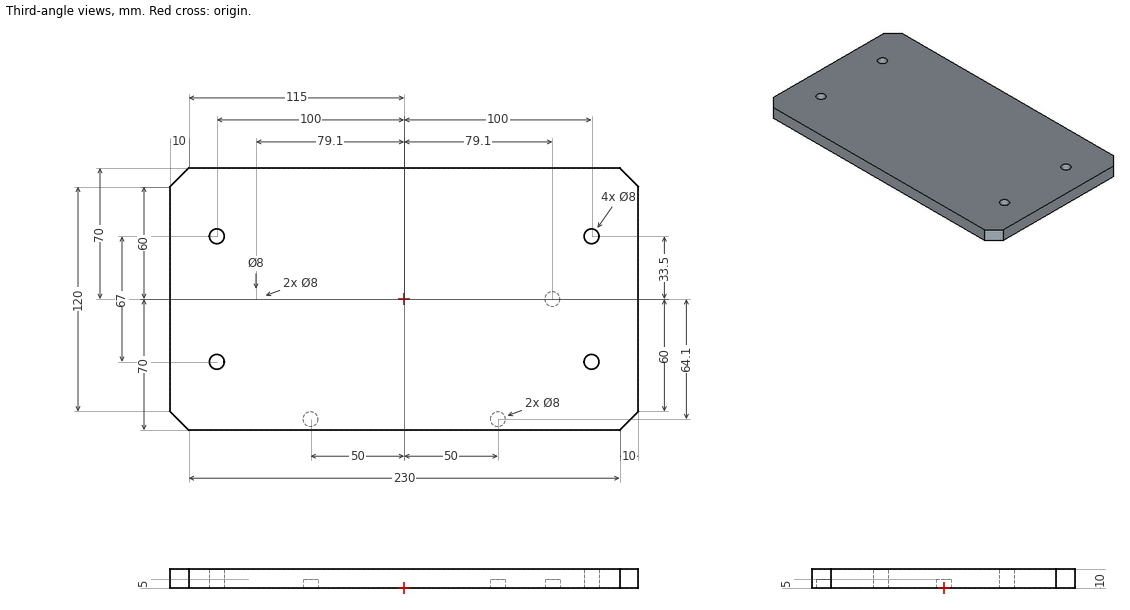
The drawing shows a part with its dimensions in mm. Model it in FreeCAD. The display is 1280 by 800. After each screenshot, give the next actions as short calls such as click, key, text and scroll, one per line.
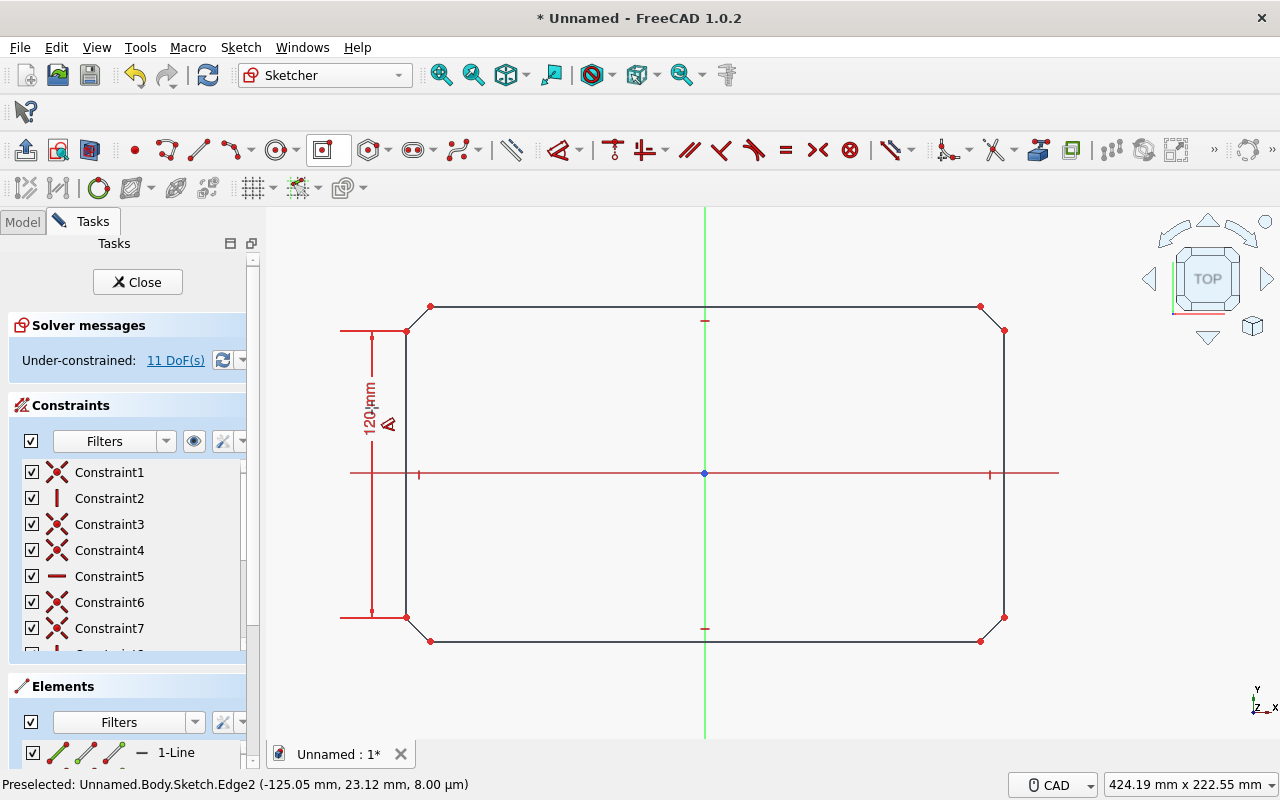
click(595, 642)
click(579, 676)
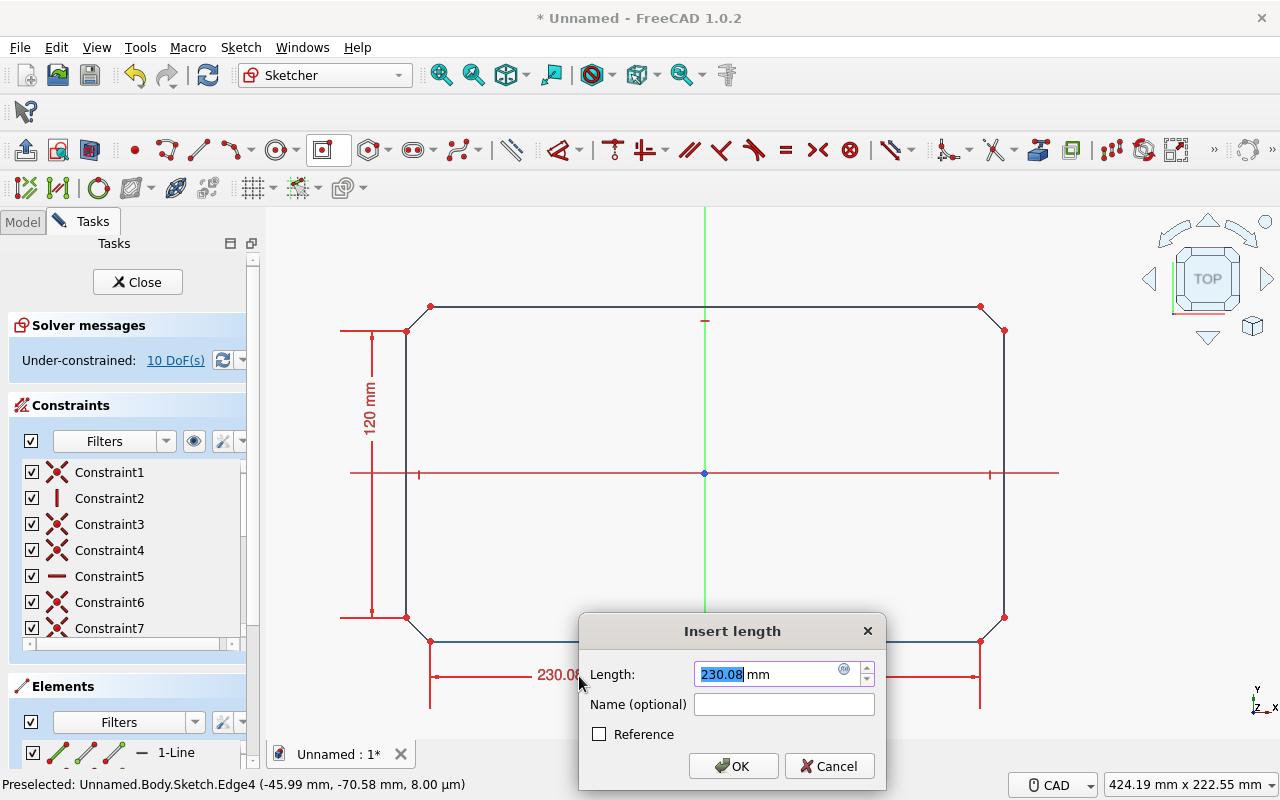
text(230)
key(Return)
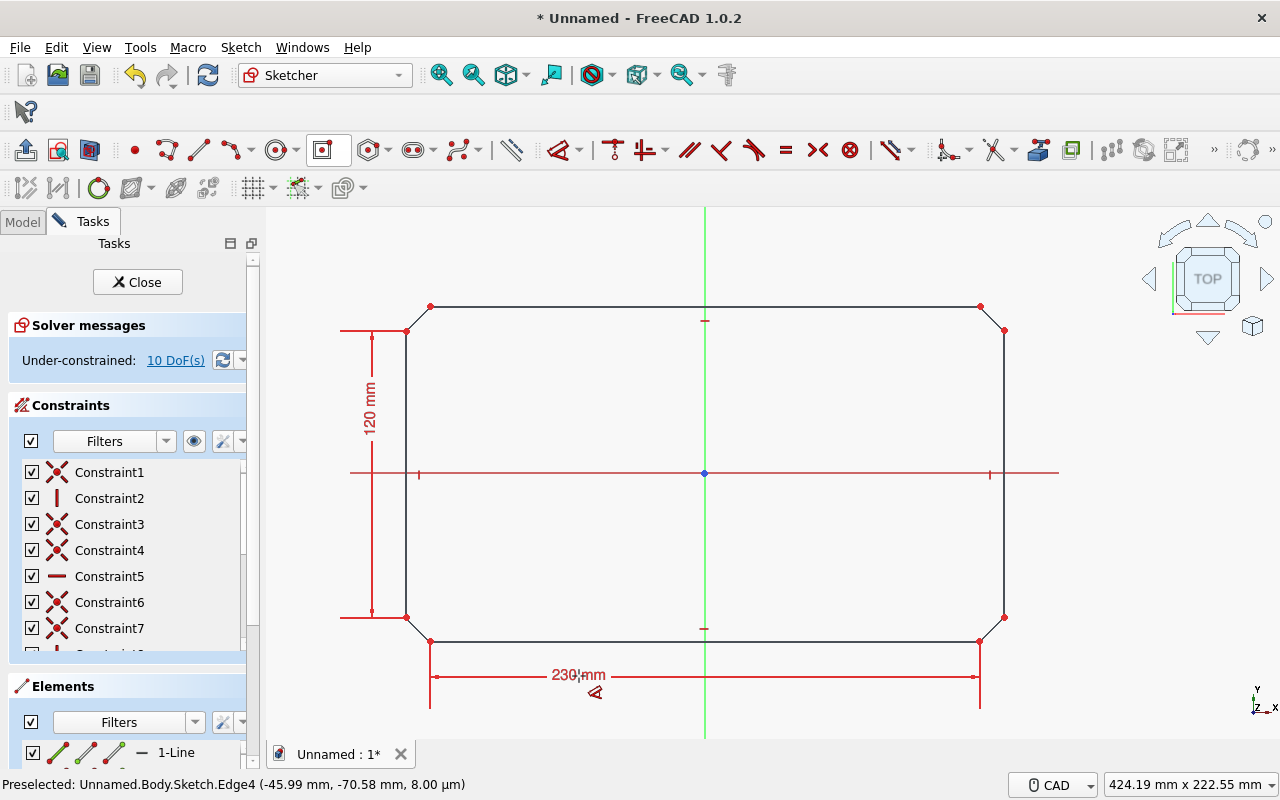
click(1004, 532)
click(1038, 408)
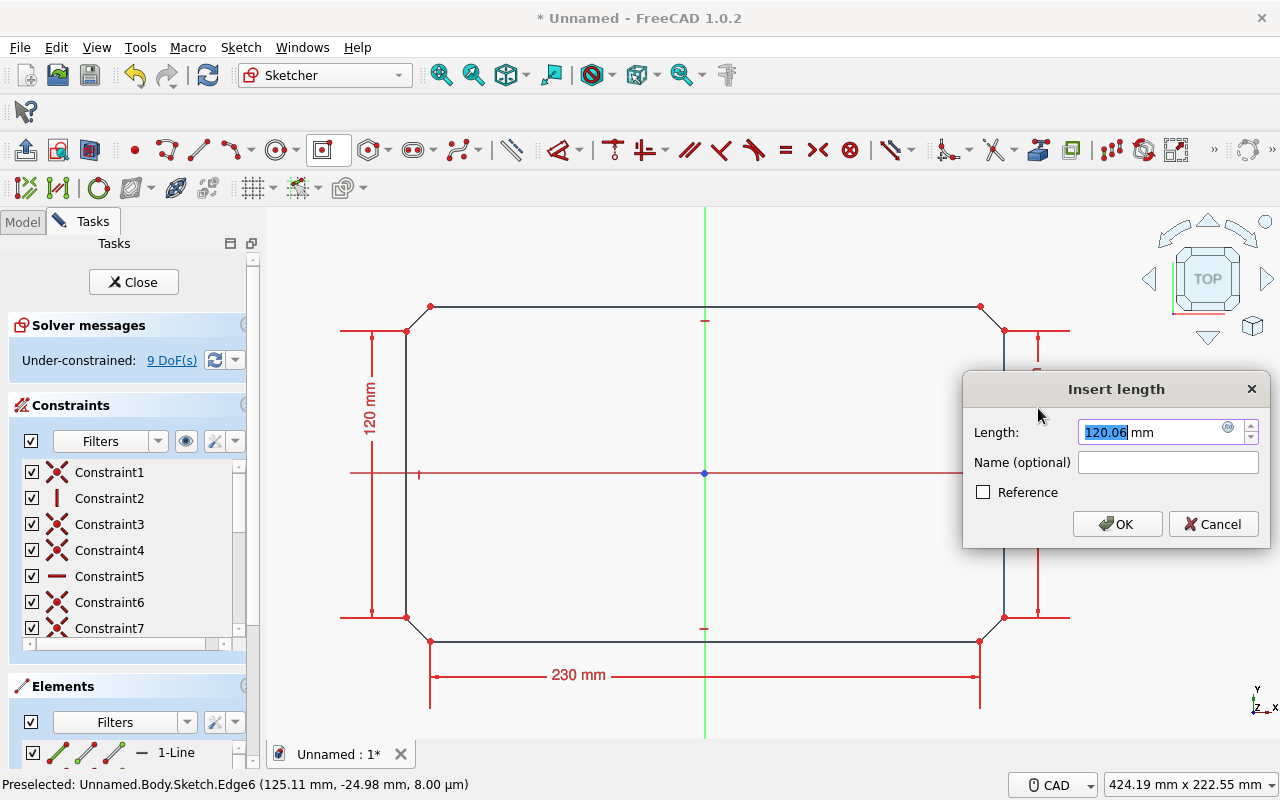
text(120)
key(Return)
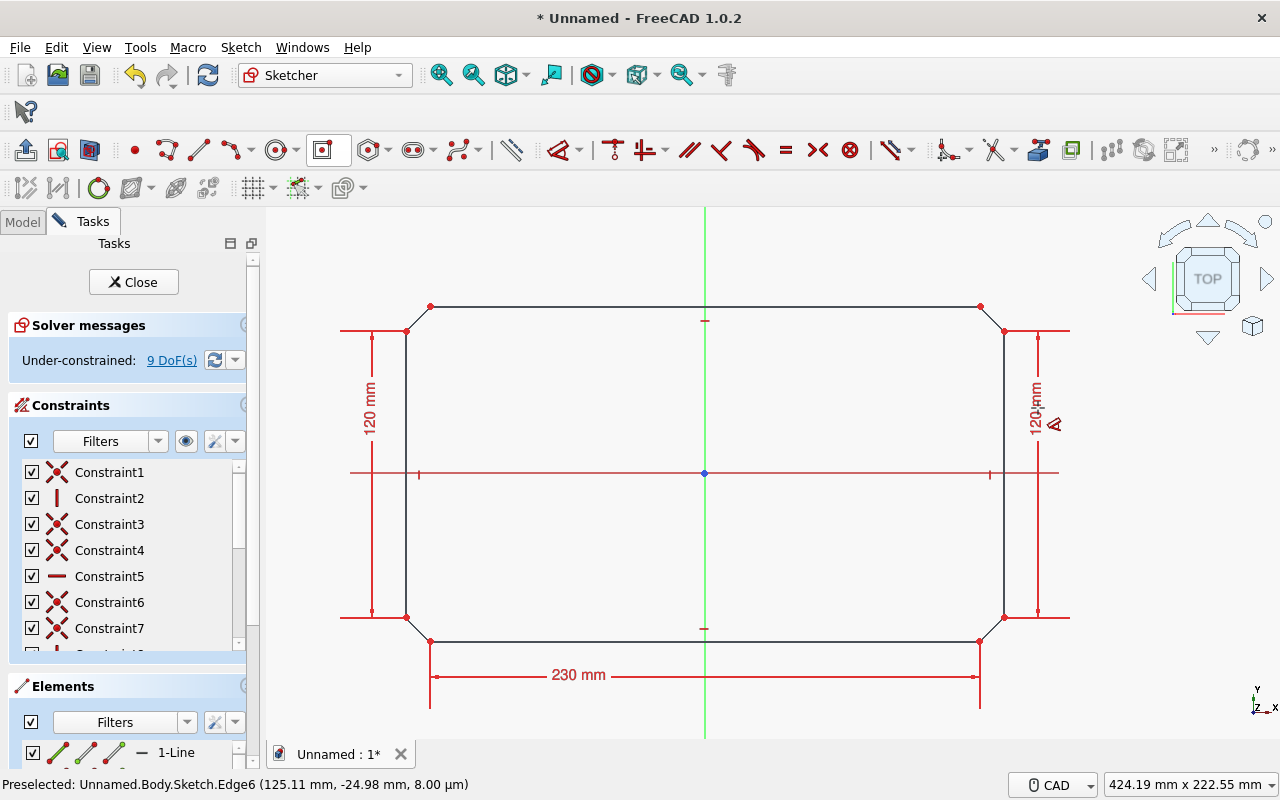
click(815, 307)
click(579, 273)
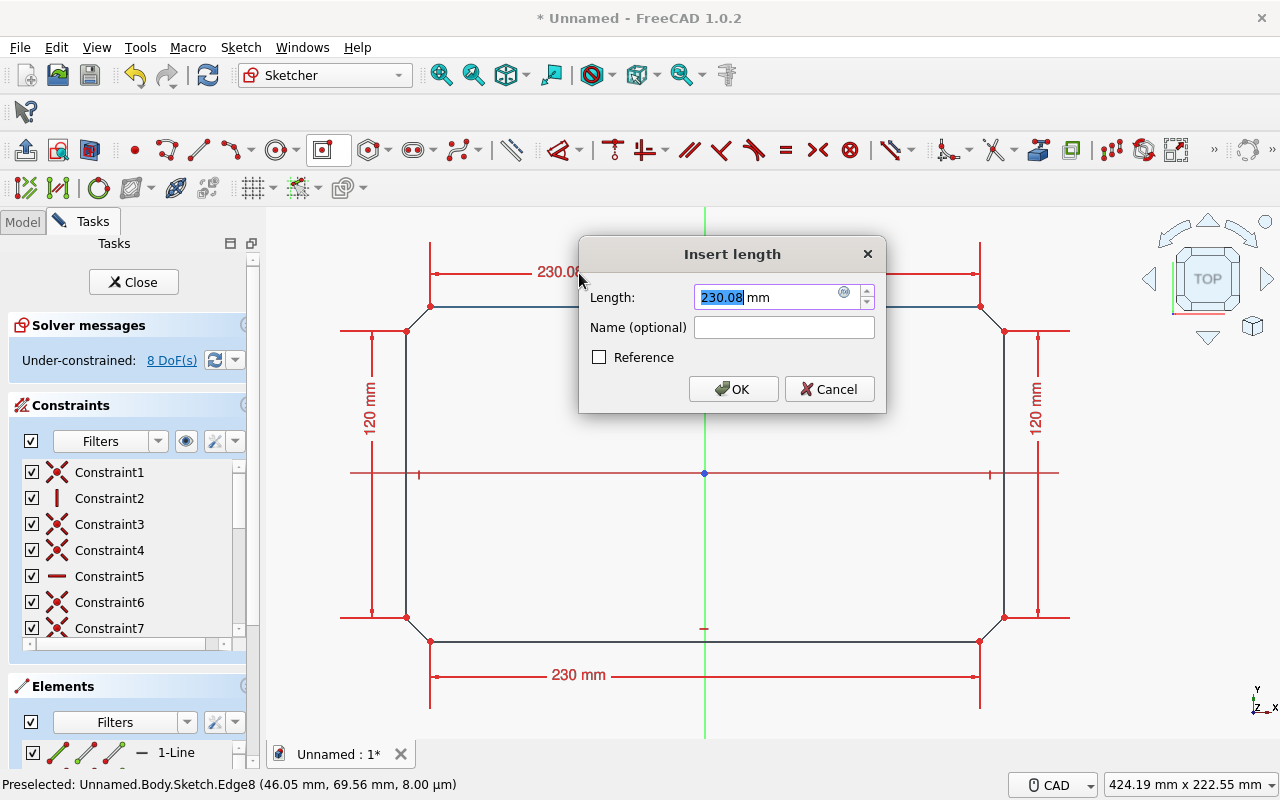
text(230)
key(Return)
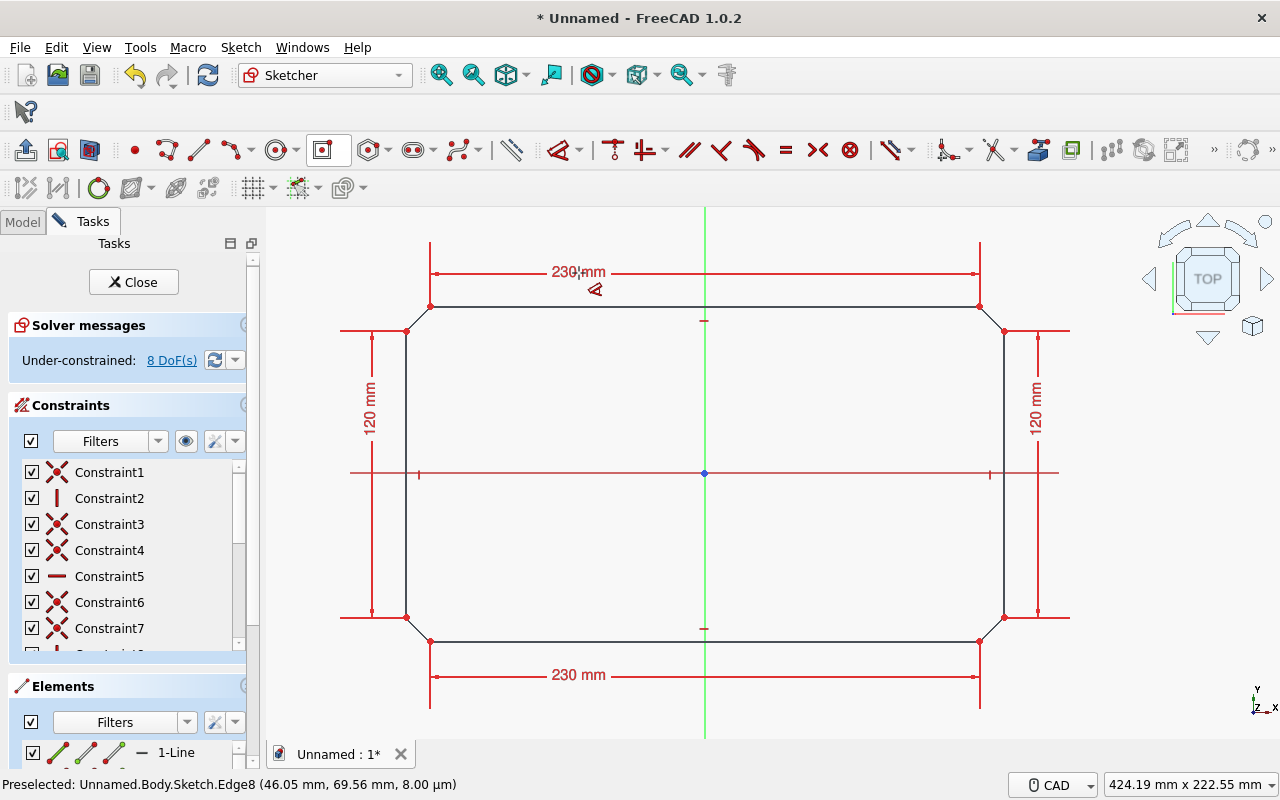
click(430, 307)
click(739, 390)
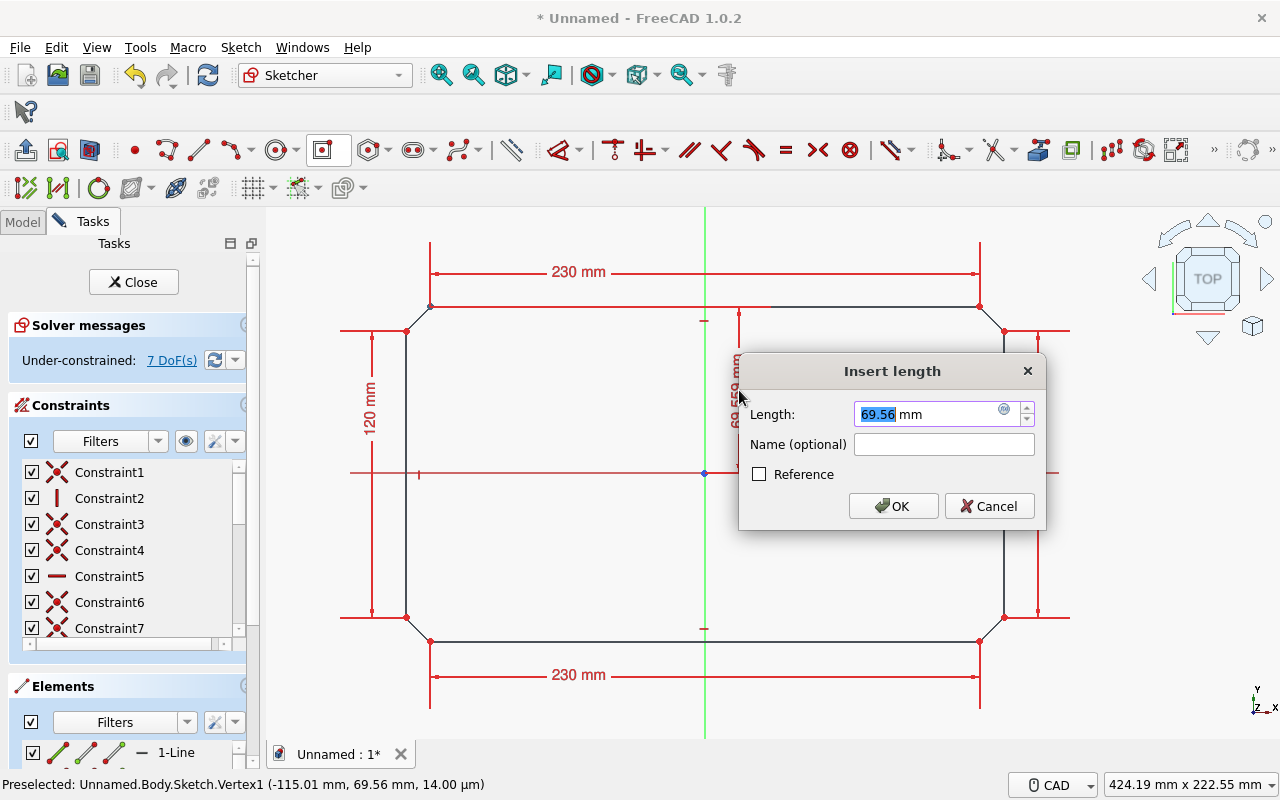
text(70)
key(Return)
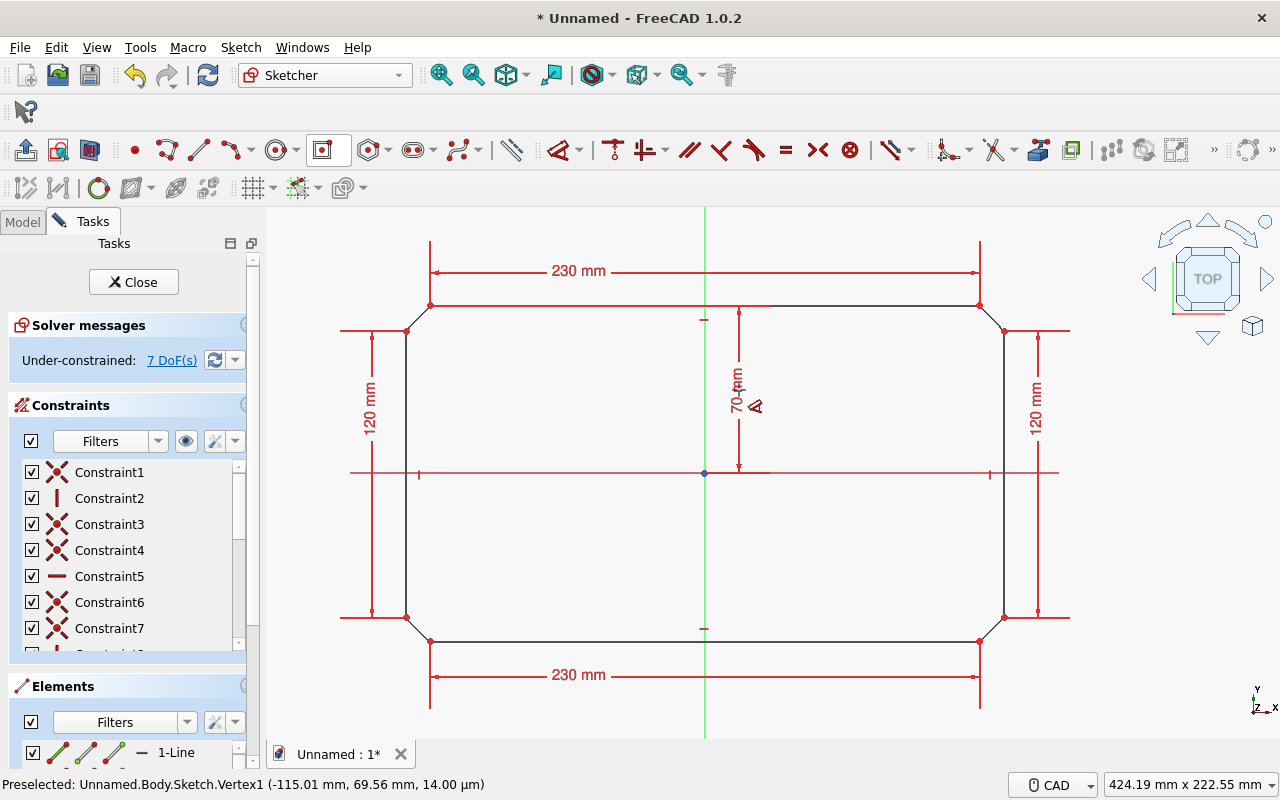
click(406, 331)
click(372, 370)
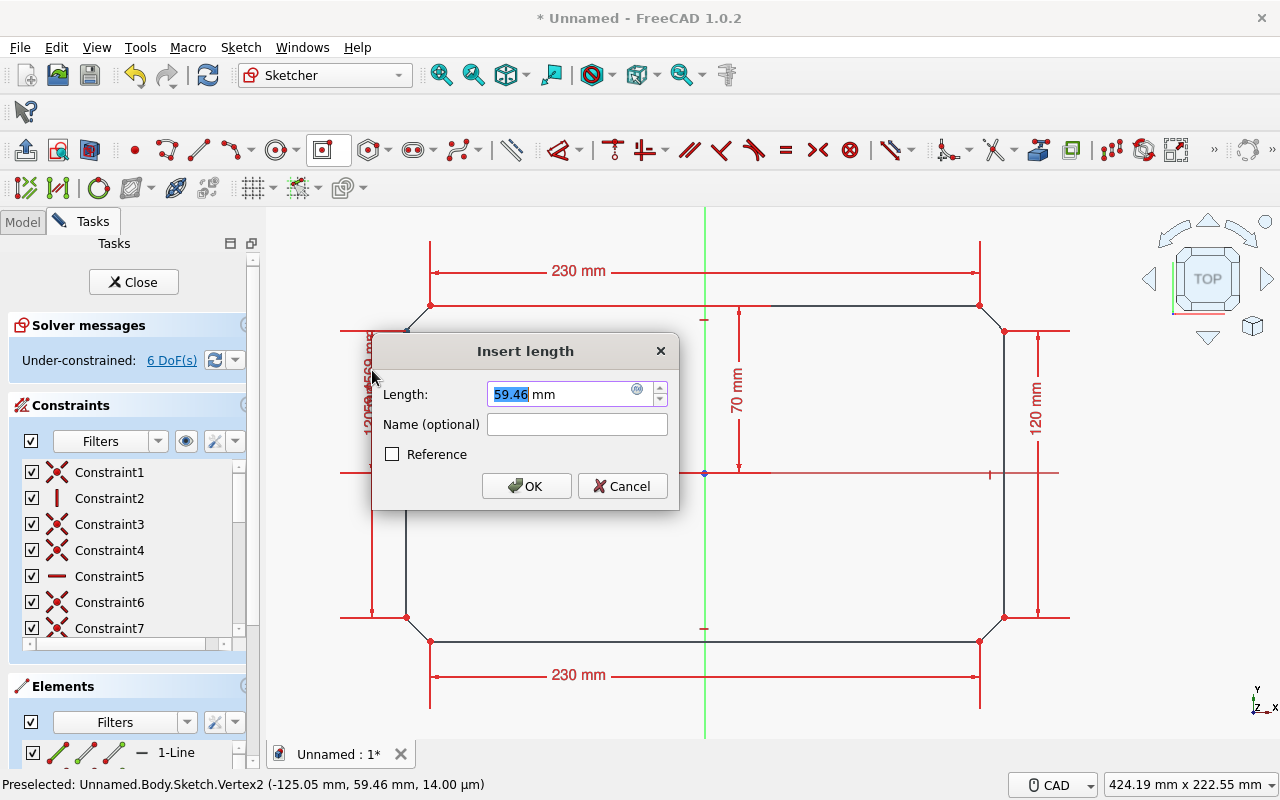
text(60)
key(Return)